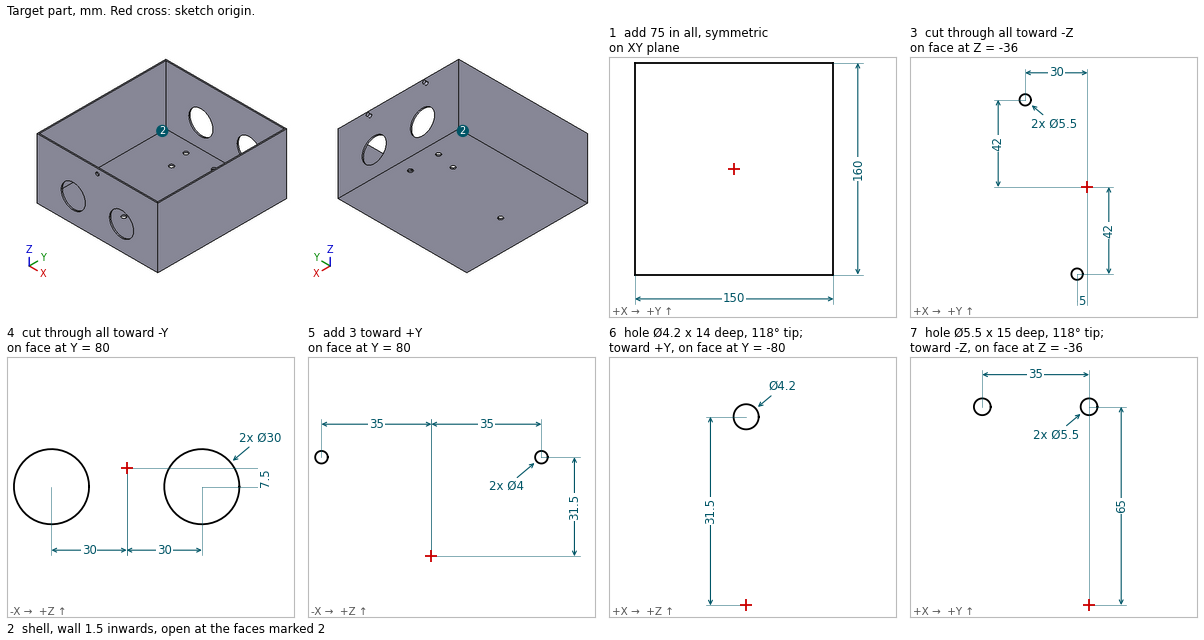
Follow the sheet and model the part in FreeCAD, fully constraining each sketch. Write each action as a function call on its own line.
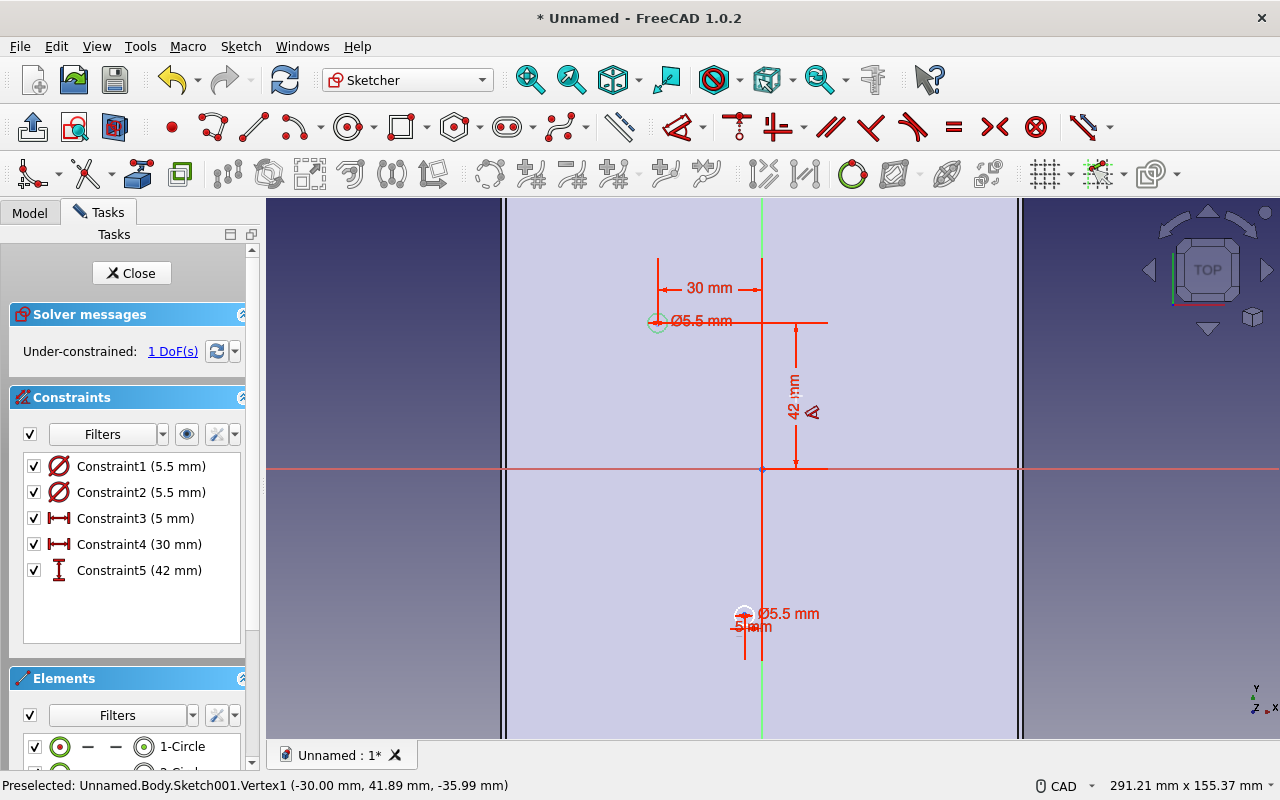
click(745, 616)
click(796, 543)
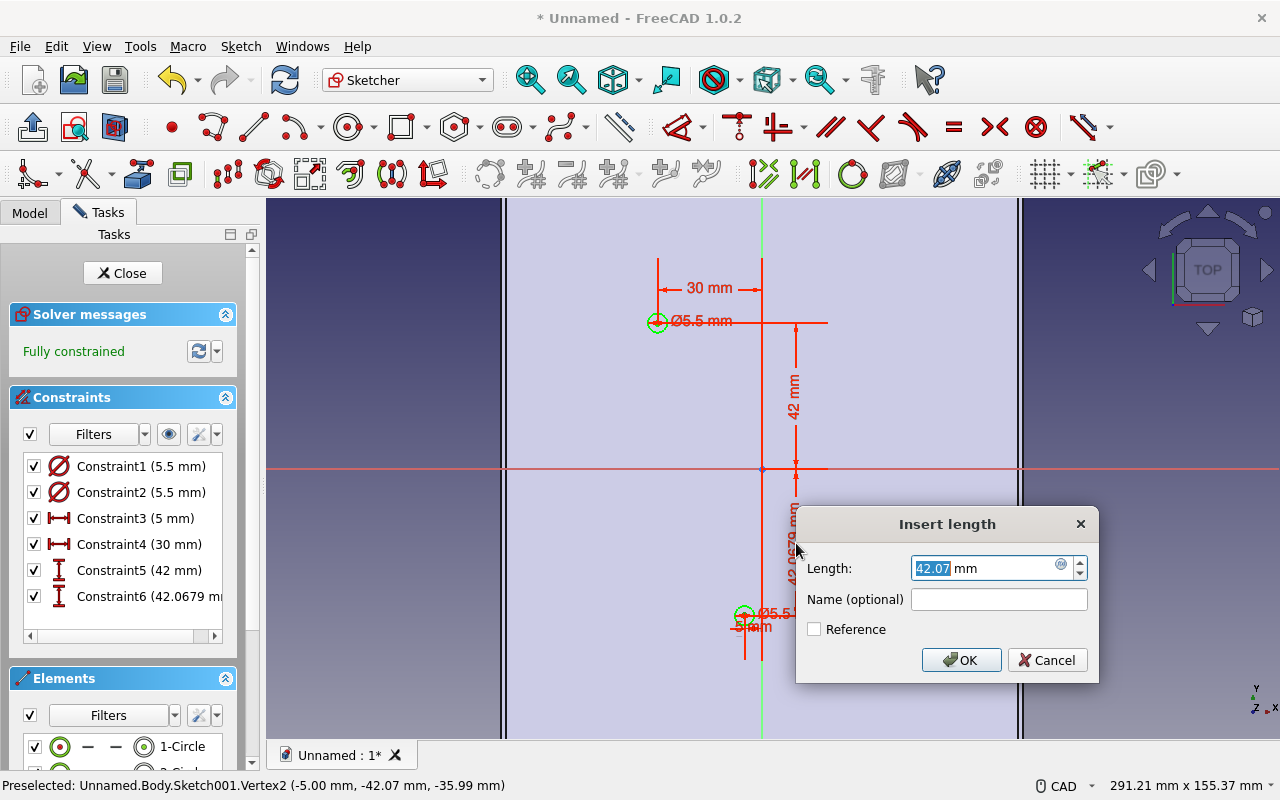
text(42)
key(Return)
key(Escape)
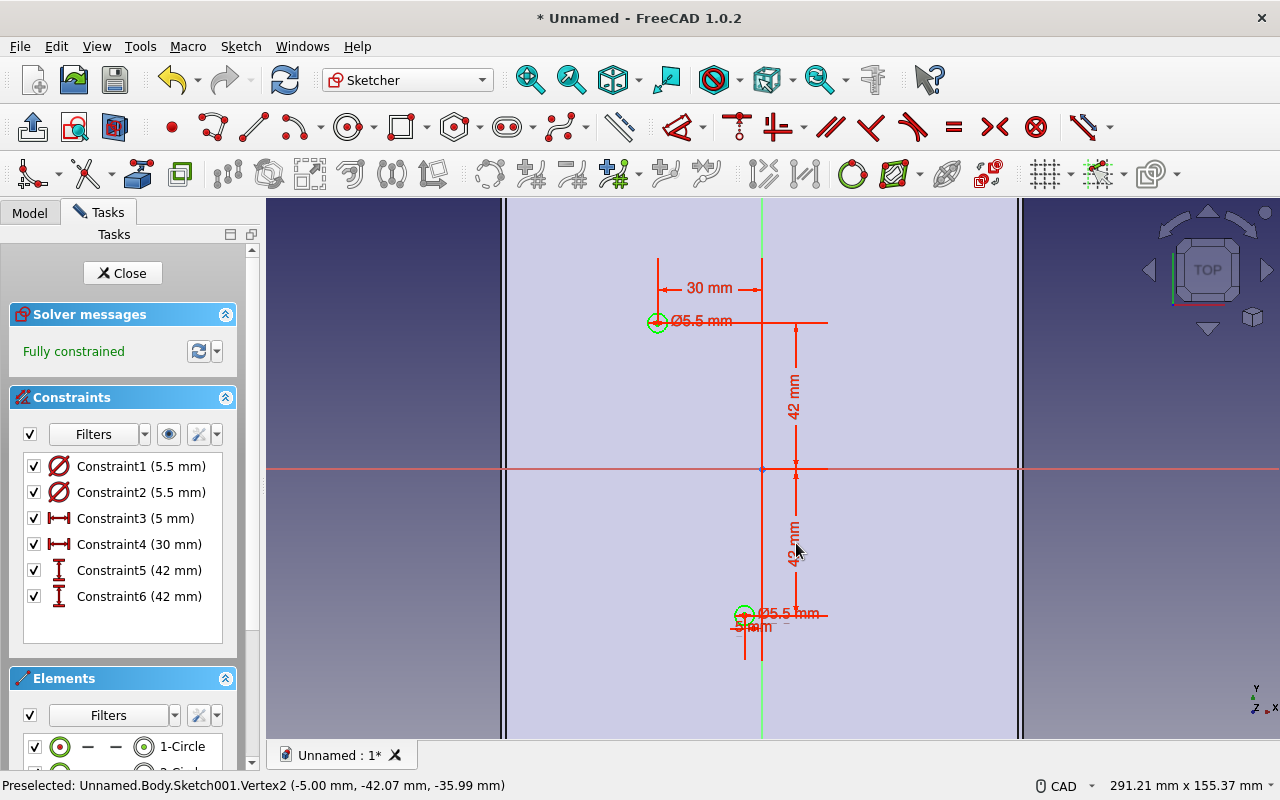
click(123, 273)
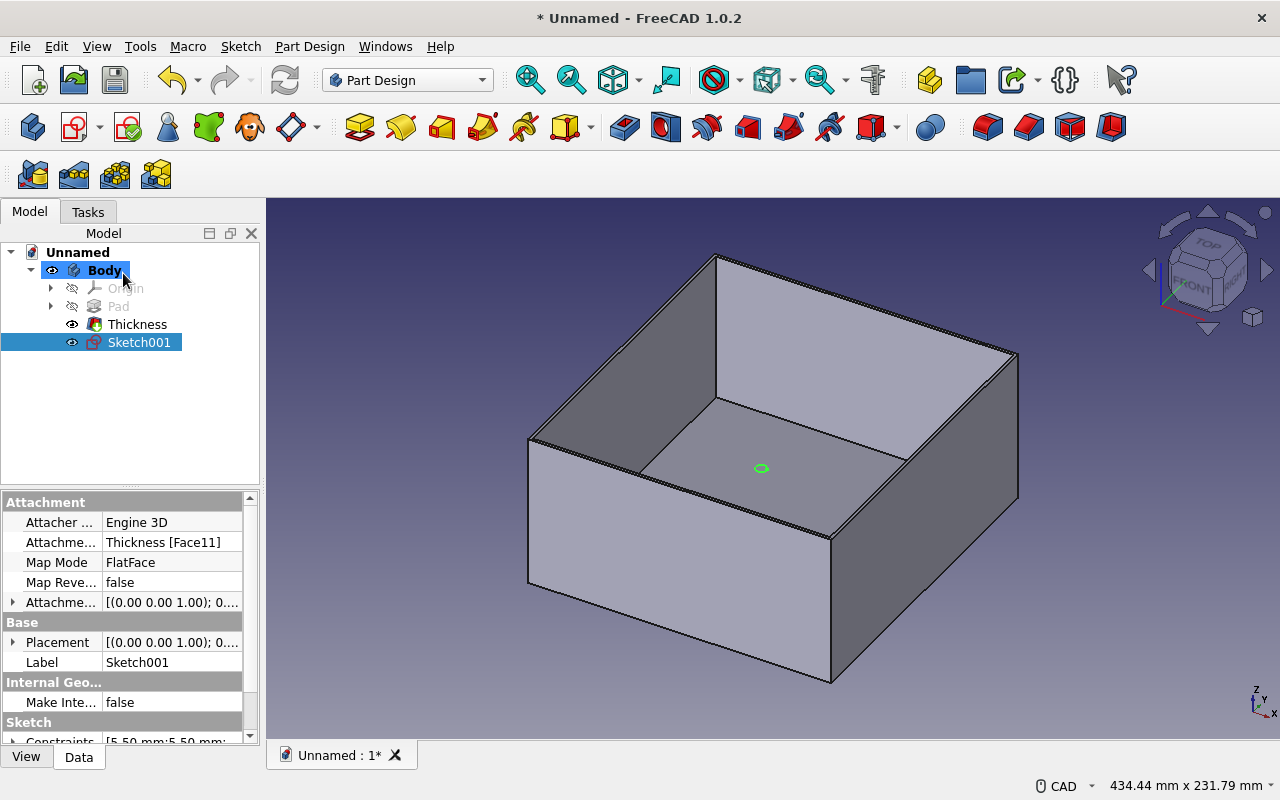
click(625, 128)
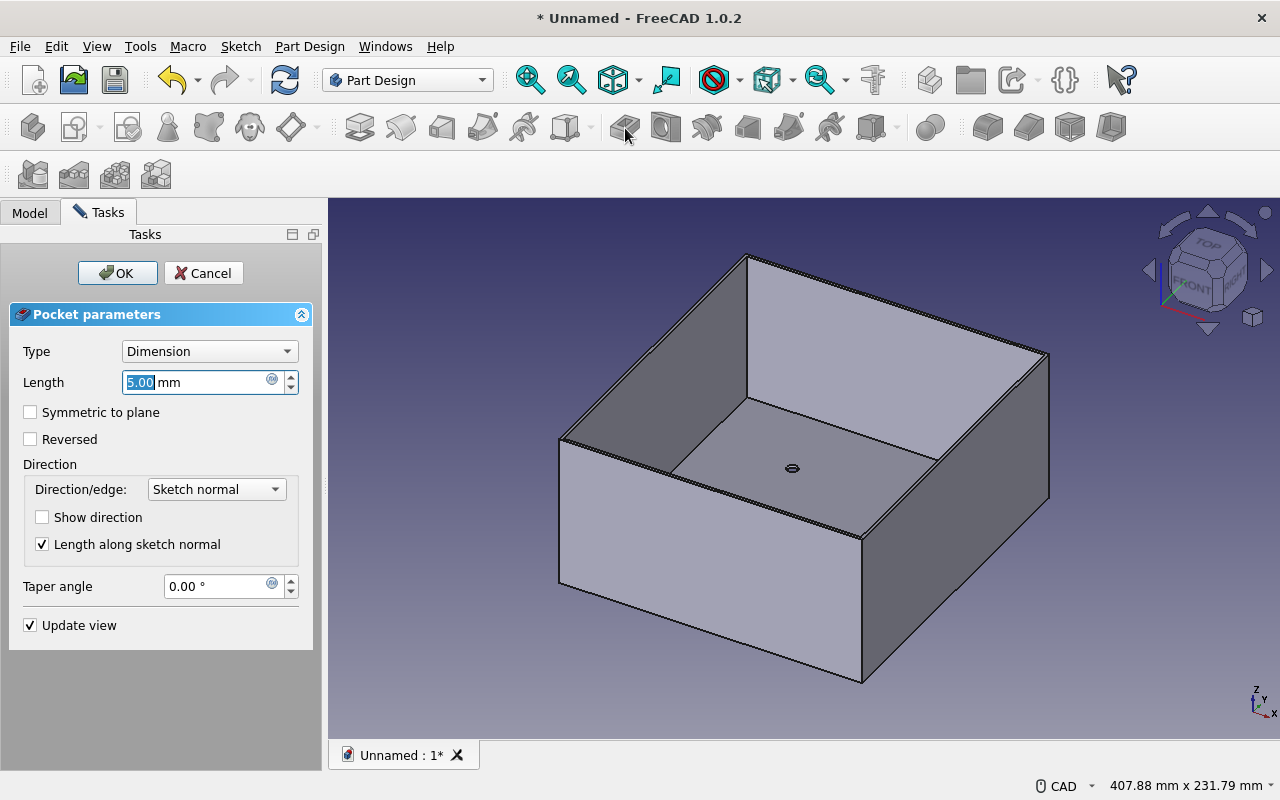
click(210, 352)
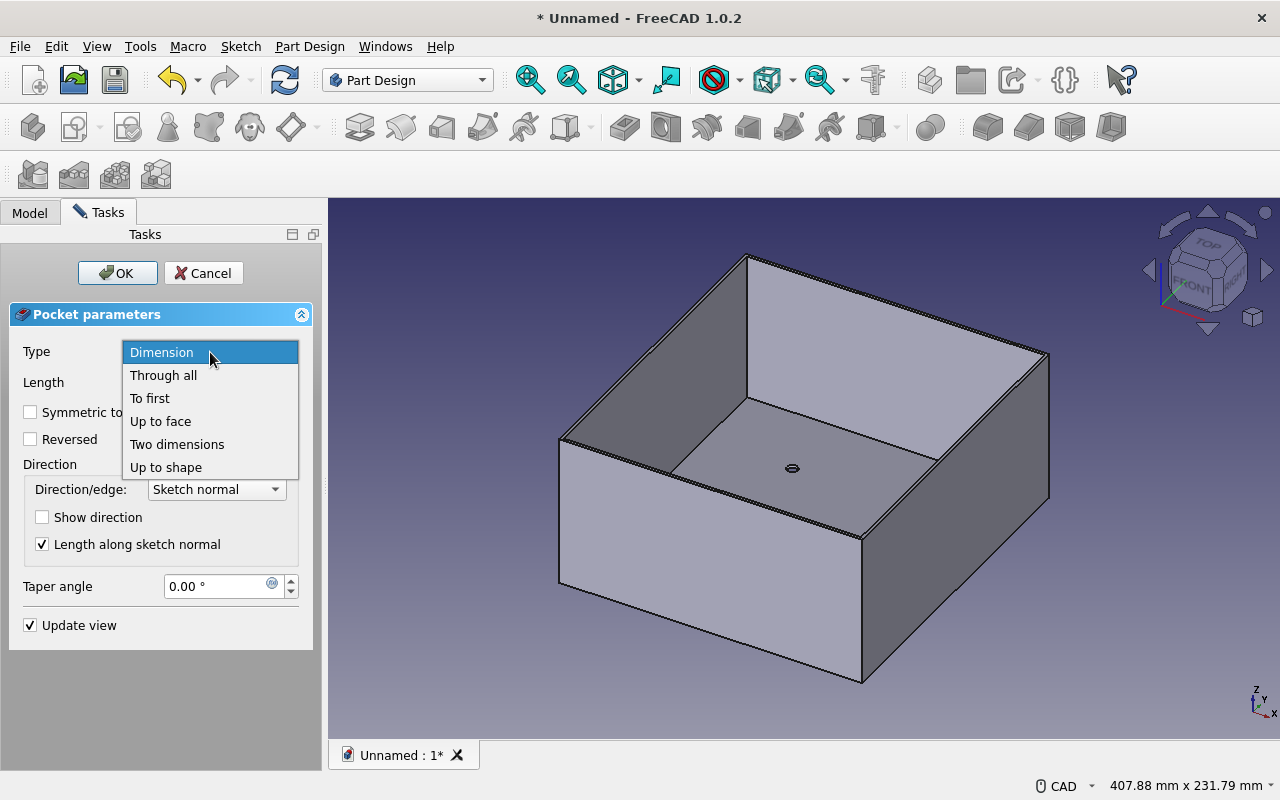
click(208, 376)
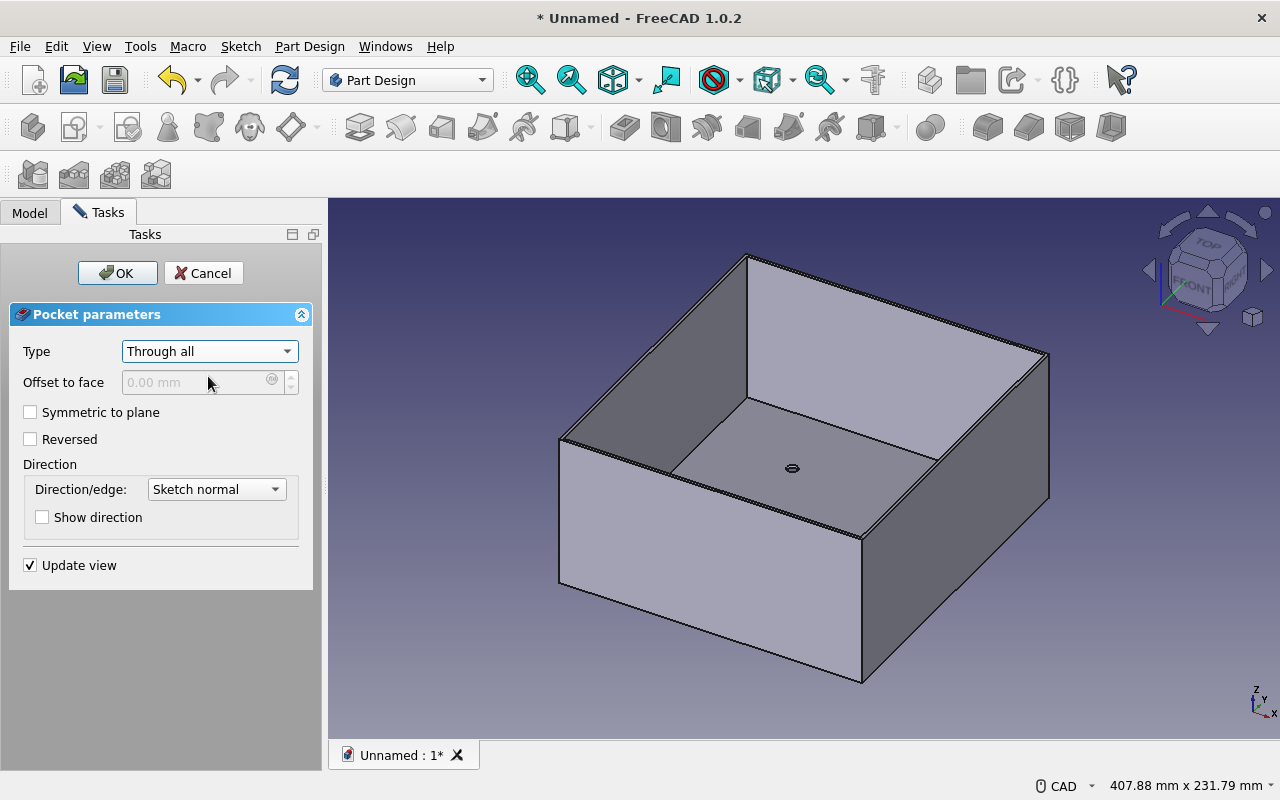
click(118, 273)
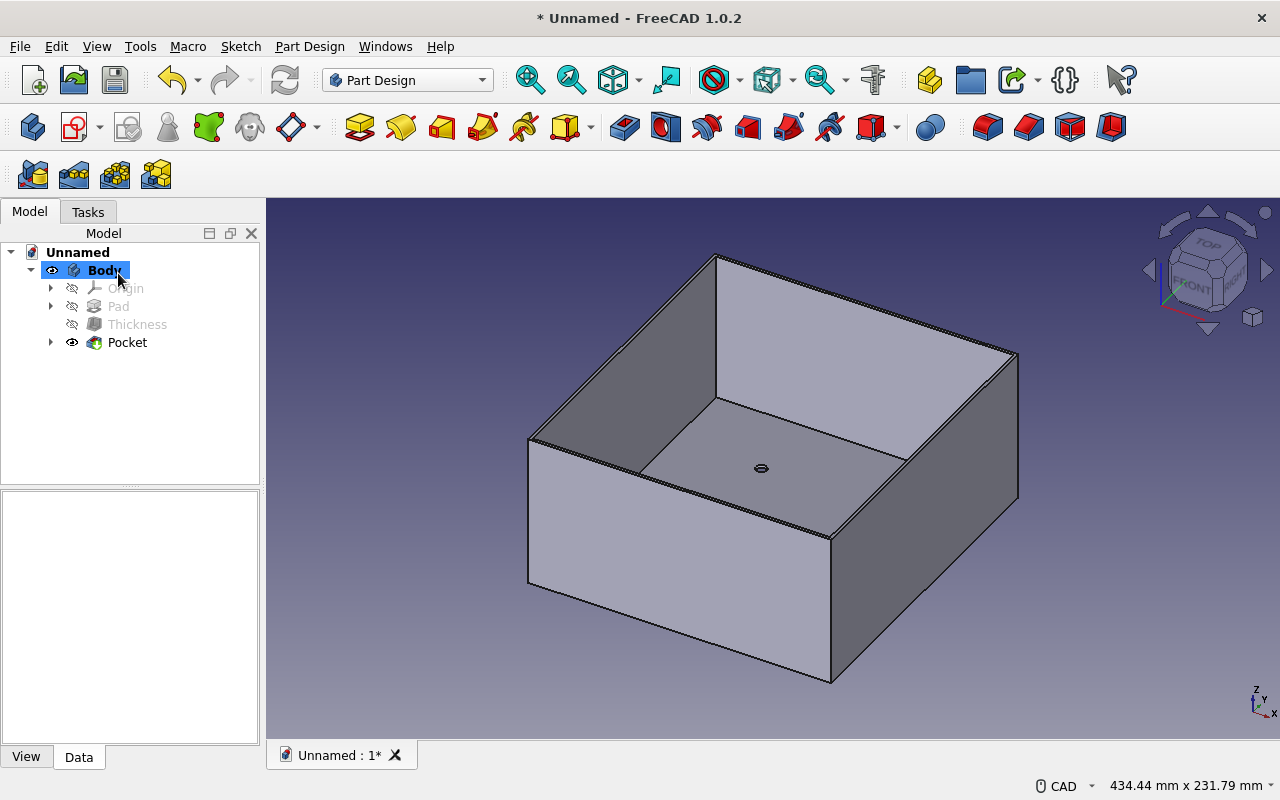
key(4)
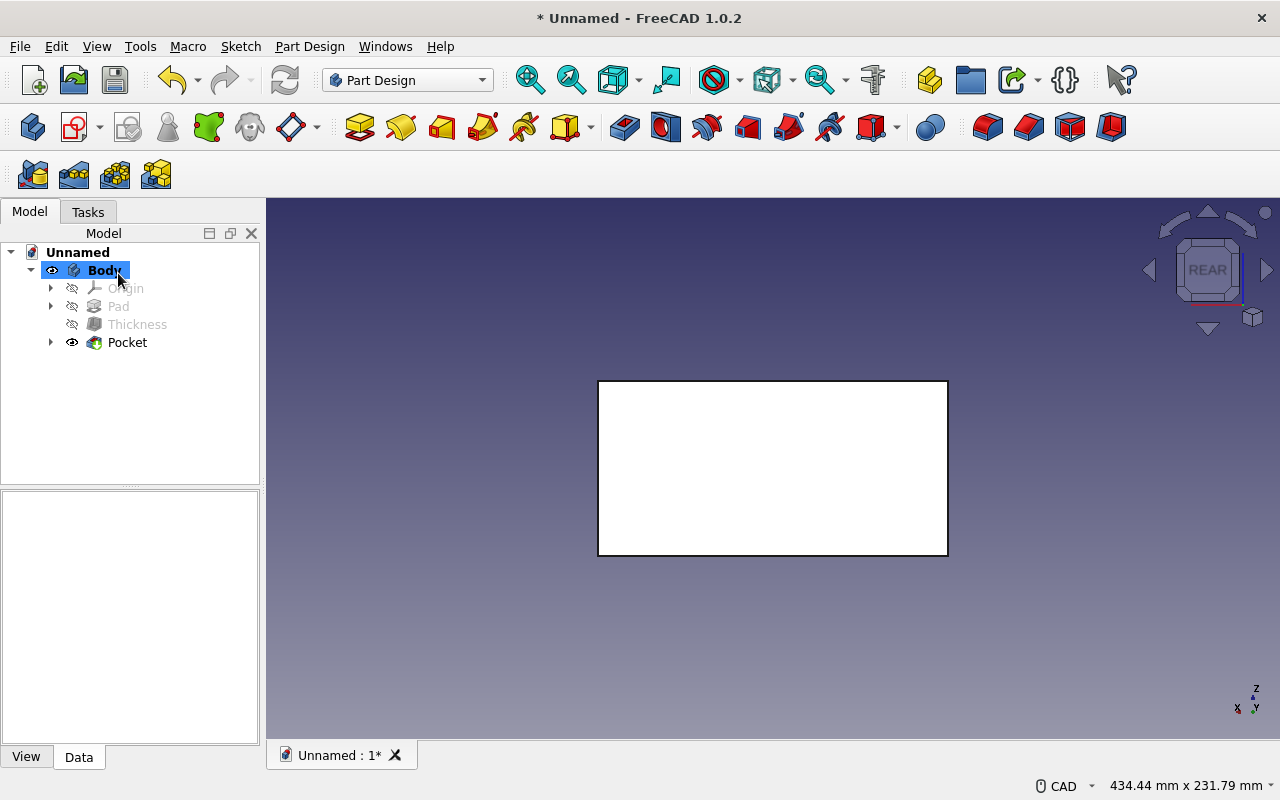
click(531, 80)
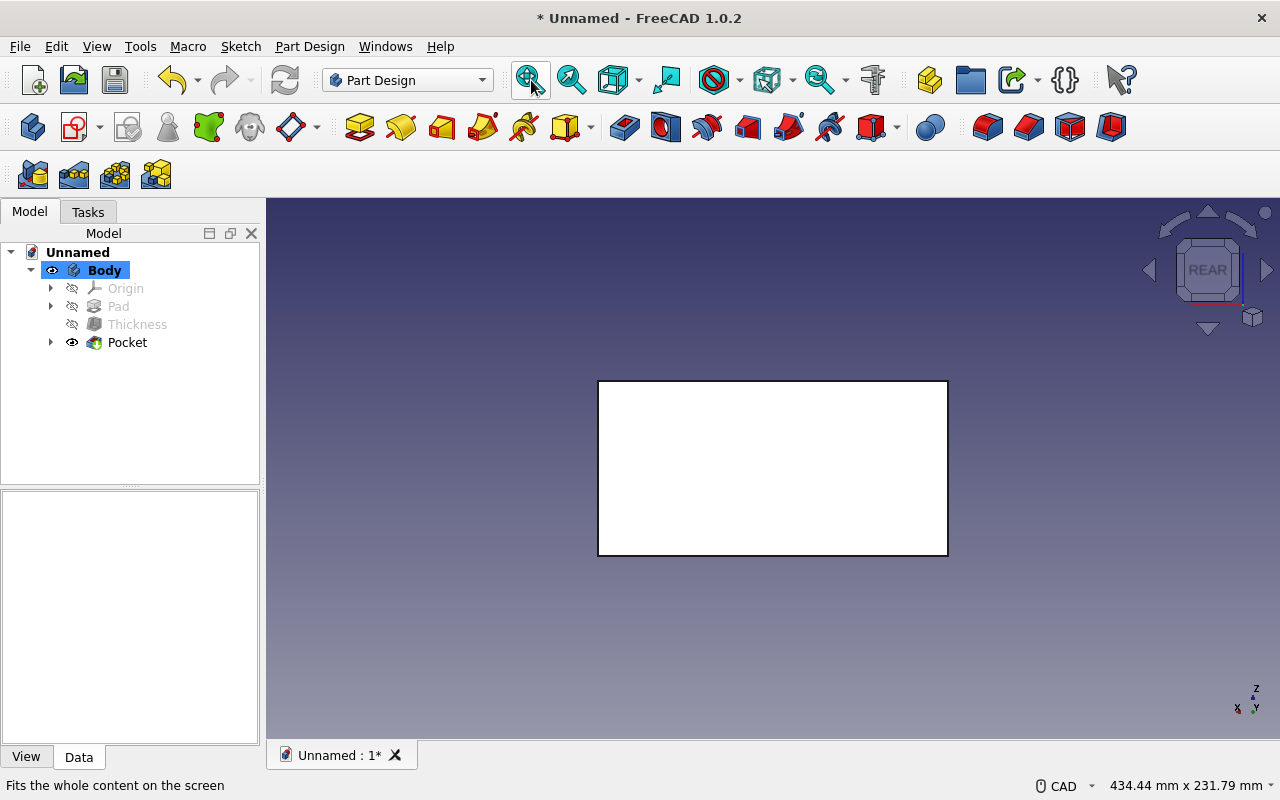
click(723, 468)